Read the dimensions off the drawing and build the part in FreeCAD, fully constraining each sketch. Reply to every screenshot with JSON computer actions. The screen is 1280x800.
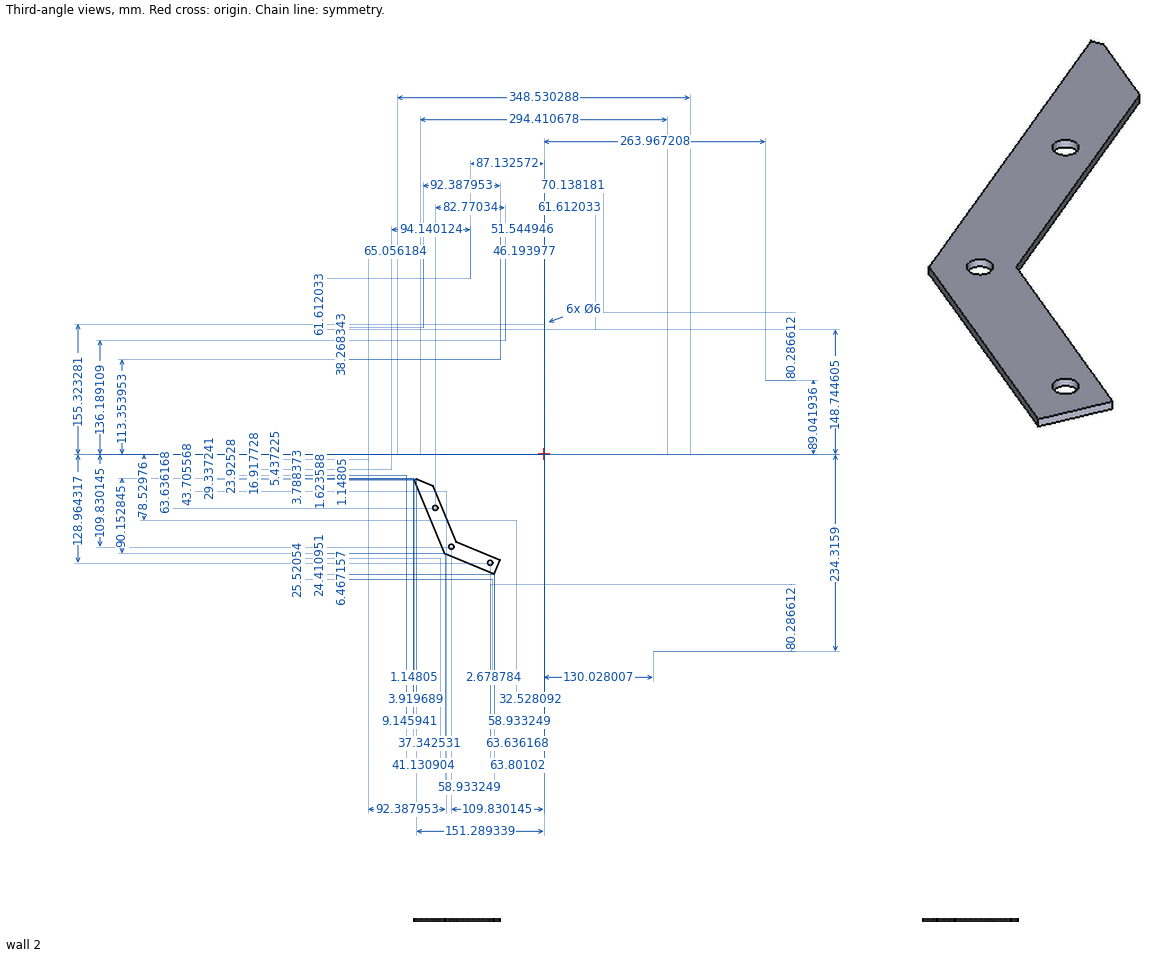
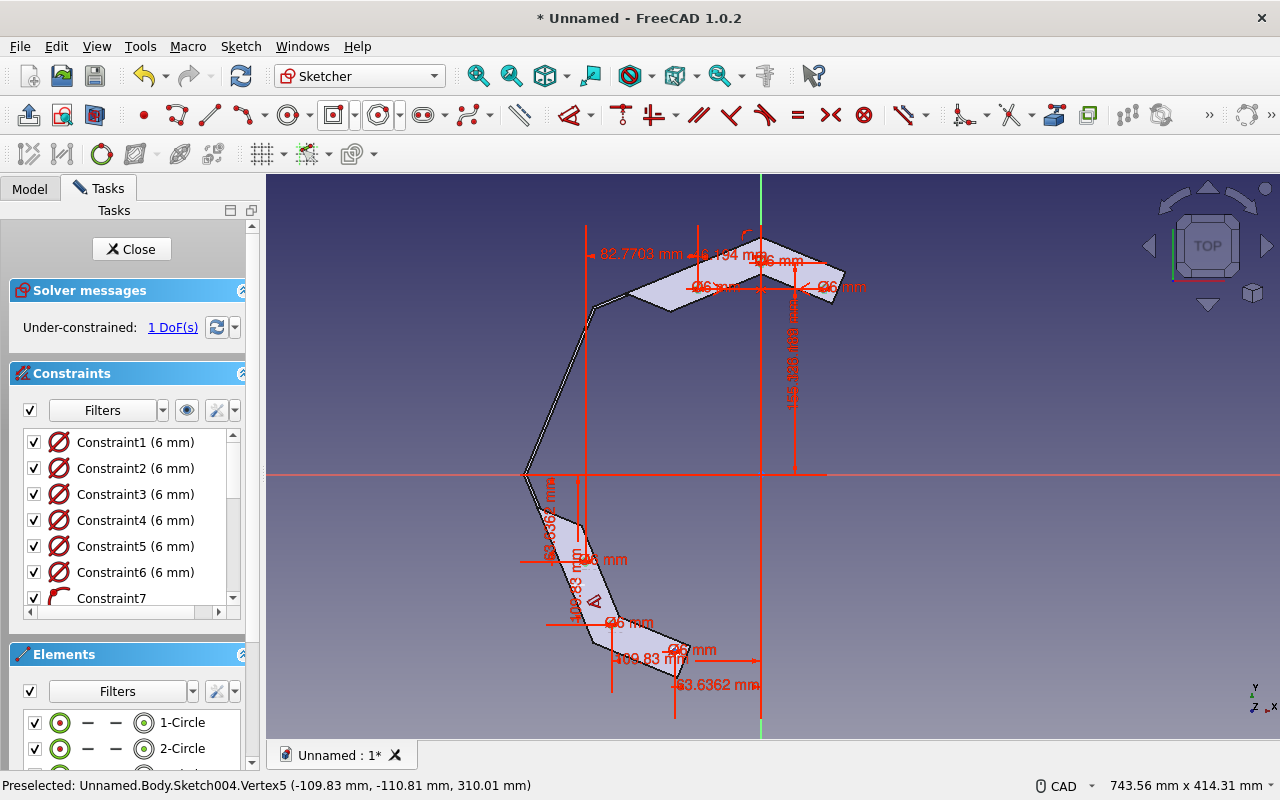
{"action": "left_click", "coordinate": [675, 652]}
{"action": "left_click", "coordinate": [795, 563]}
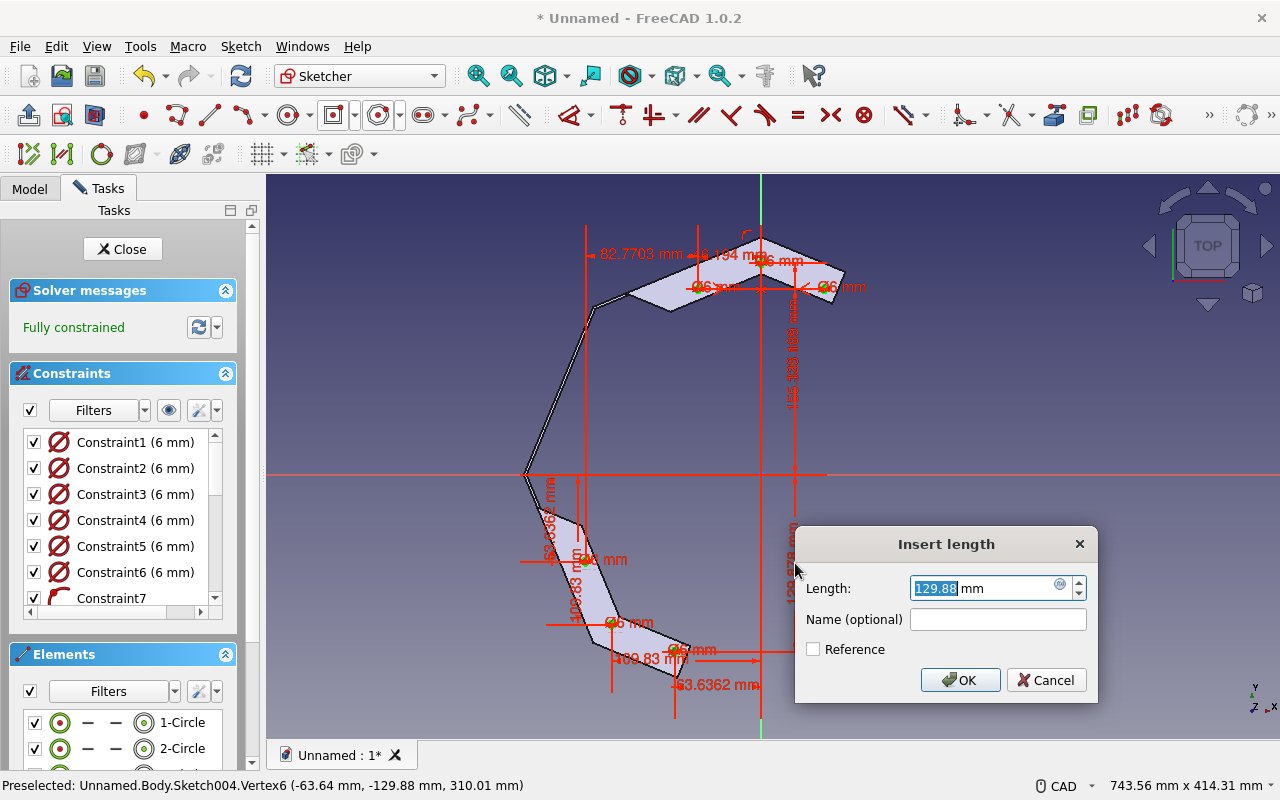
{"action": "type", "text": "128.964317"}
{"action": "key", "text": "Return"}
{"action": "key", "text": "Escape"}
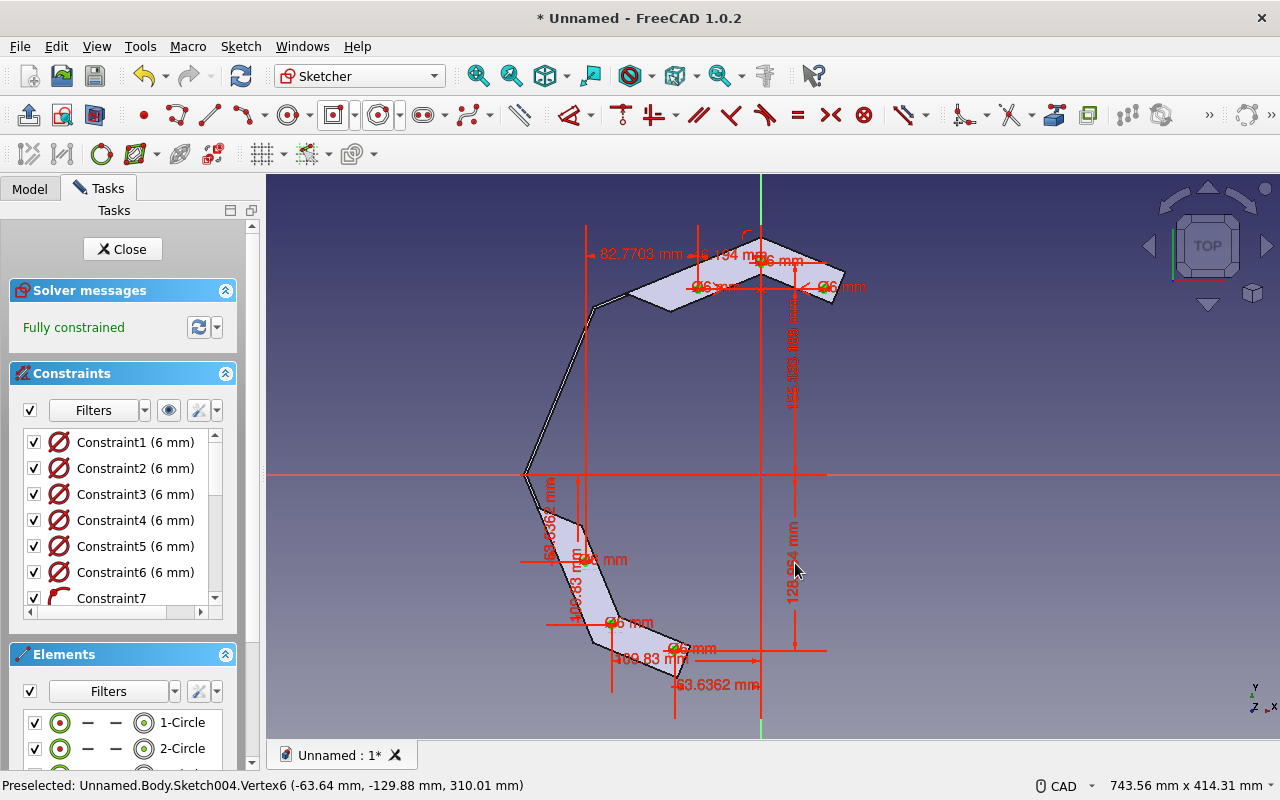
{"action": "left_click", "coordinate": [123, 249]}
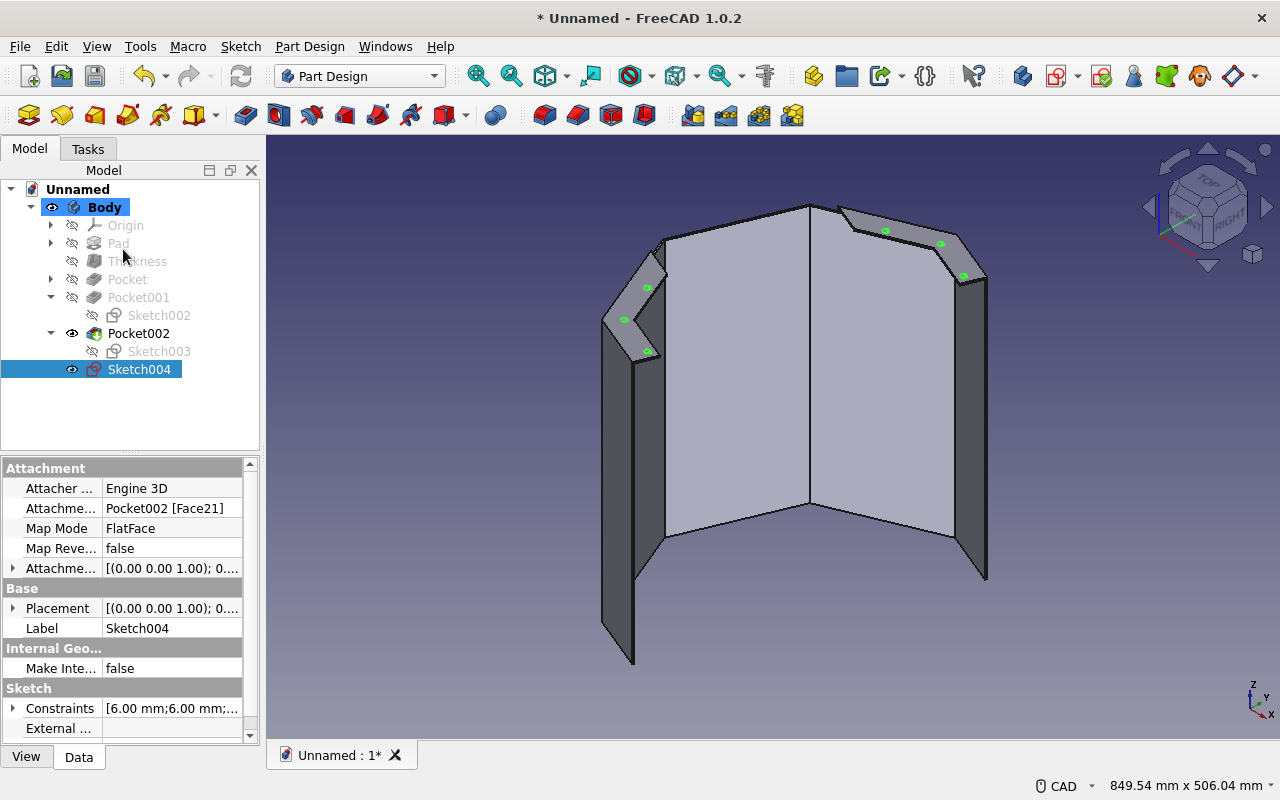
{"action": "left_click", "coordinate": [246, 116]}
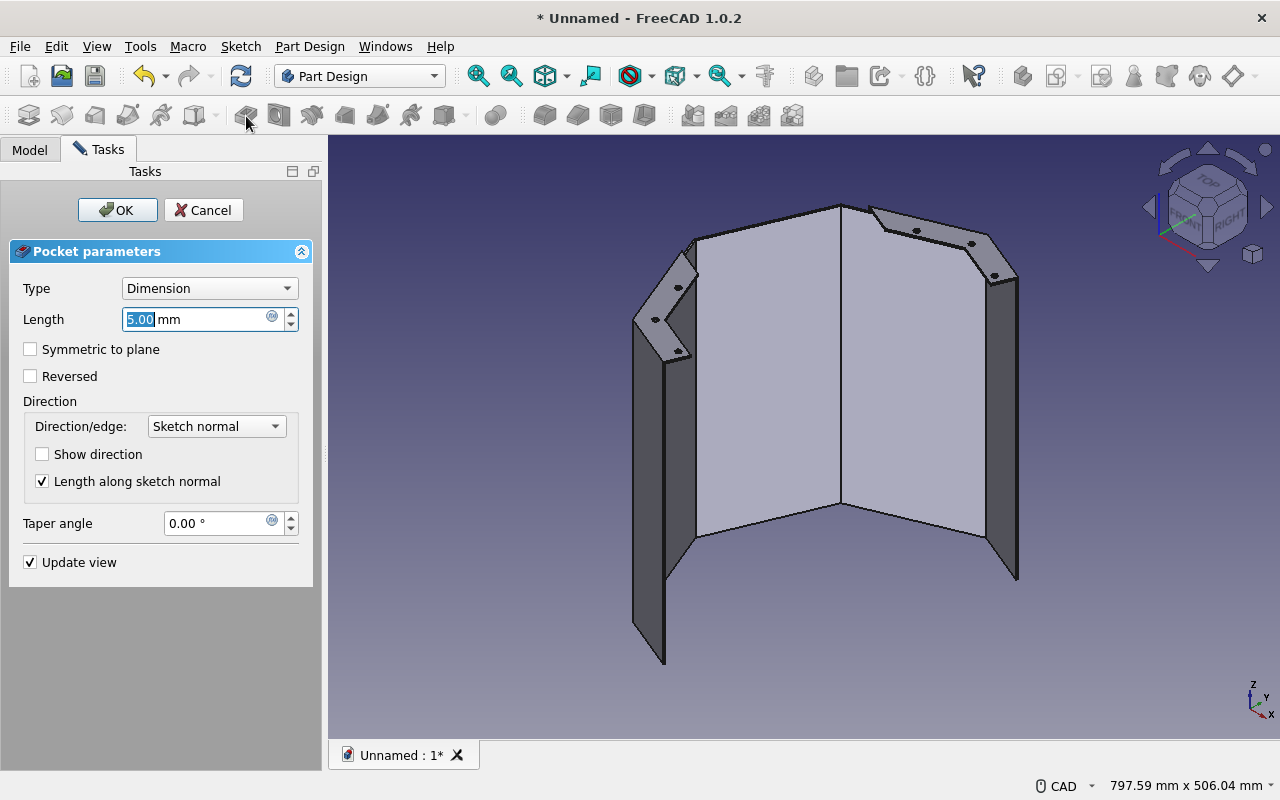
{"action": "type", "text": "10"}
{"action": "key", "text": "Tab"}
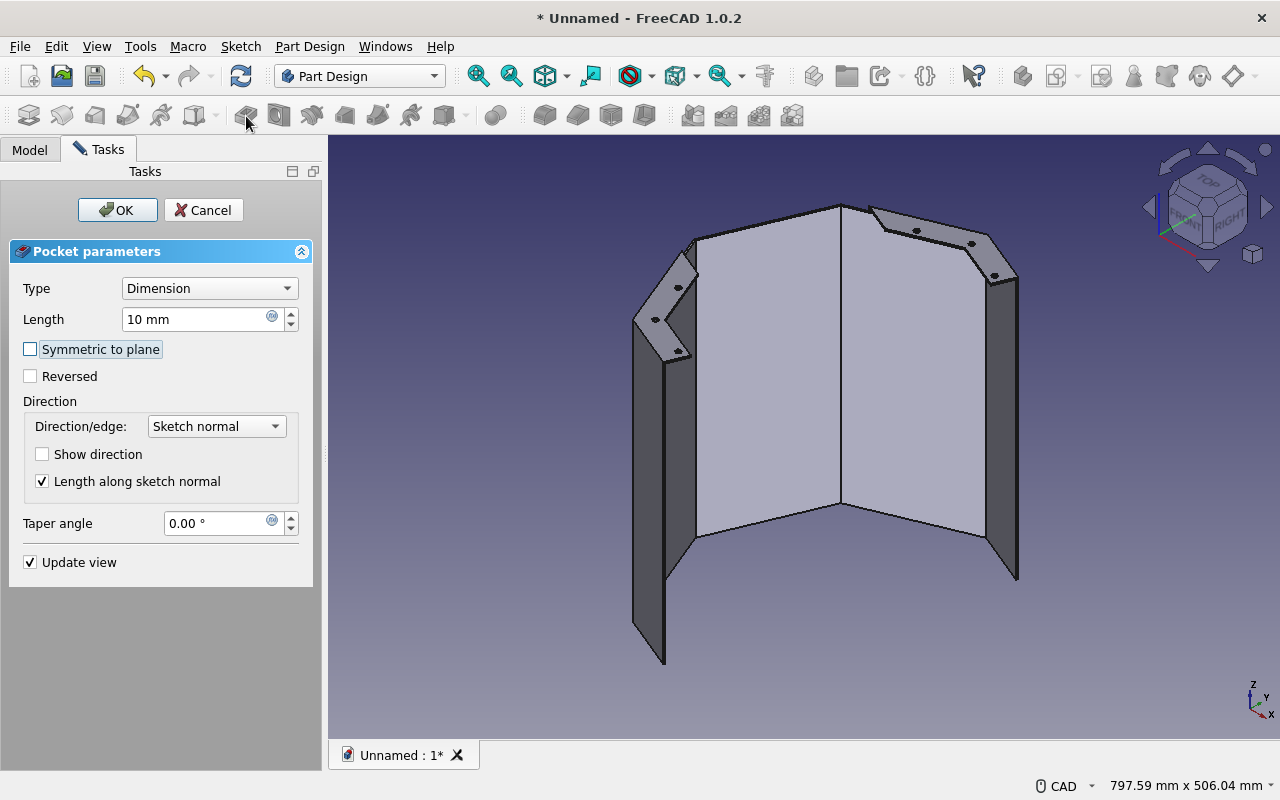
{"action": "left_click", "coordinate": [118, 210]}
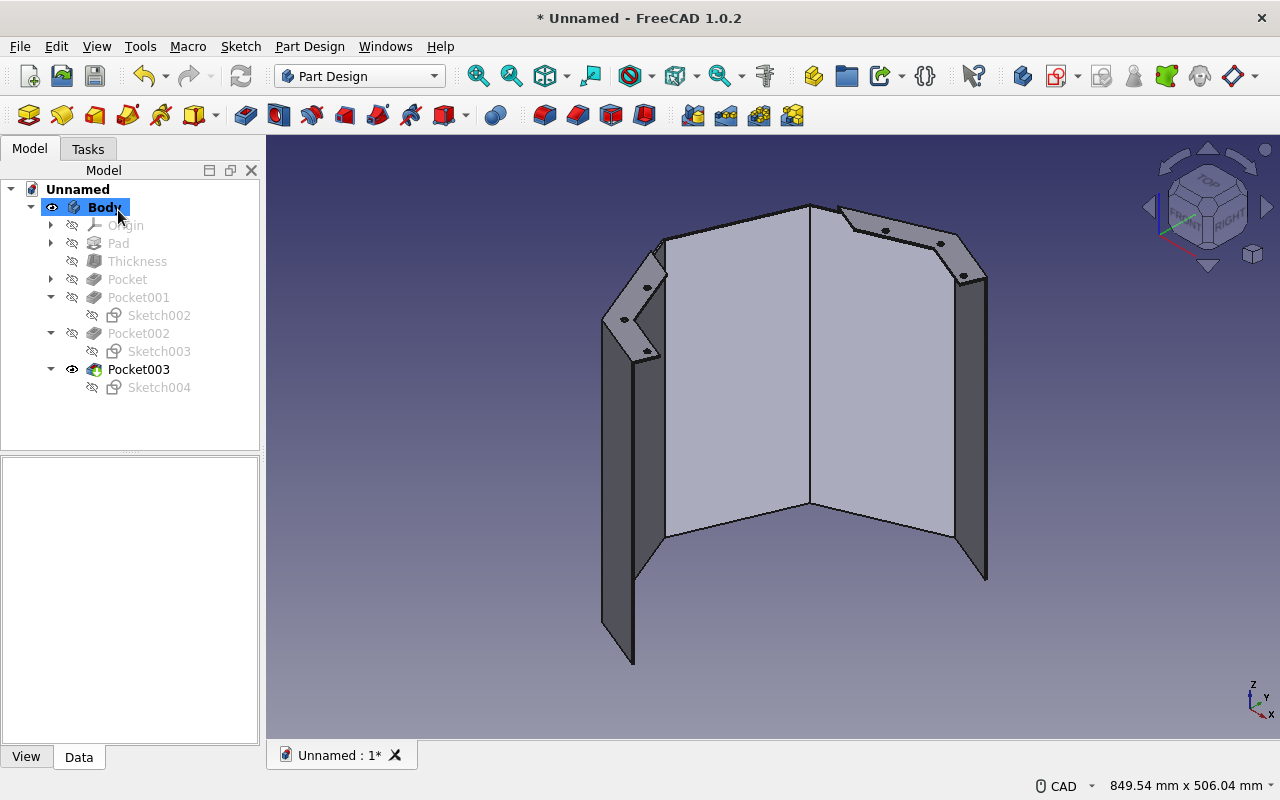
{"action": "left_click", "coordinate": [924, 234]}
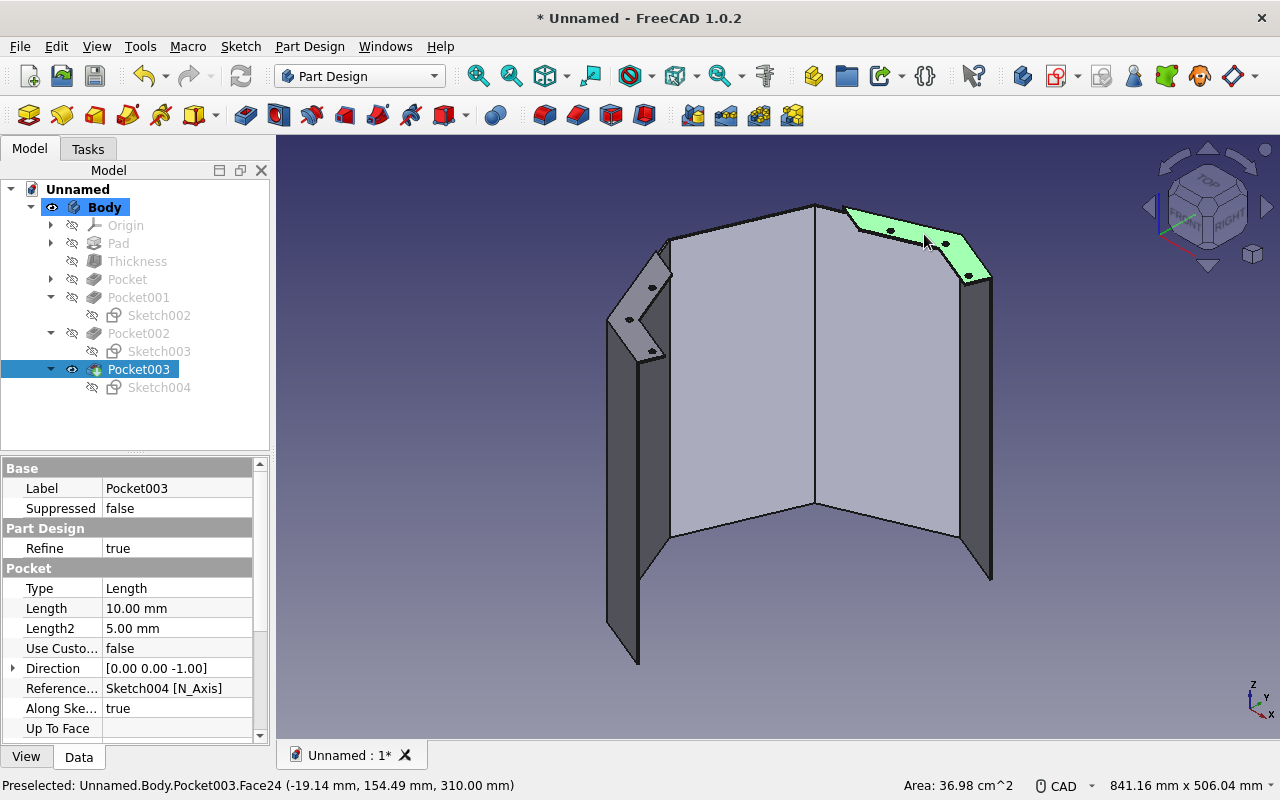
{"action": "left_click", "coordinate": [1056, 76]}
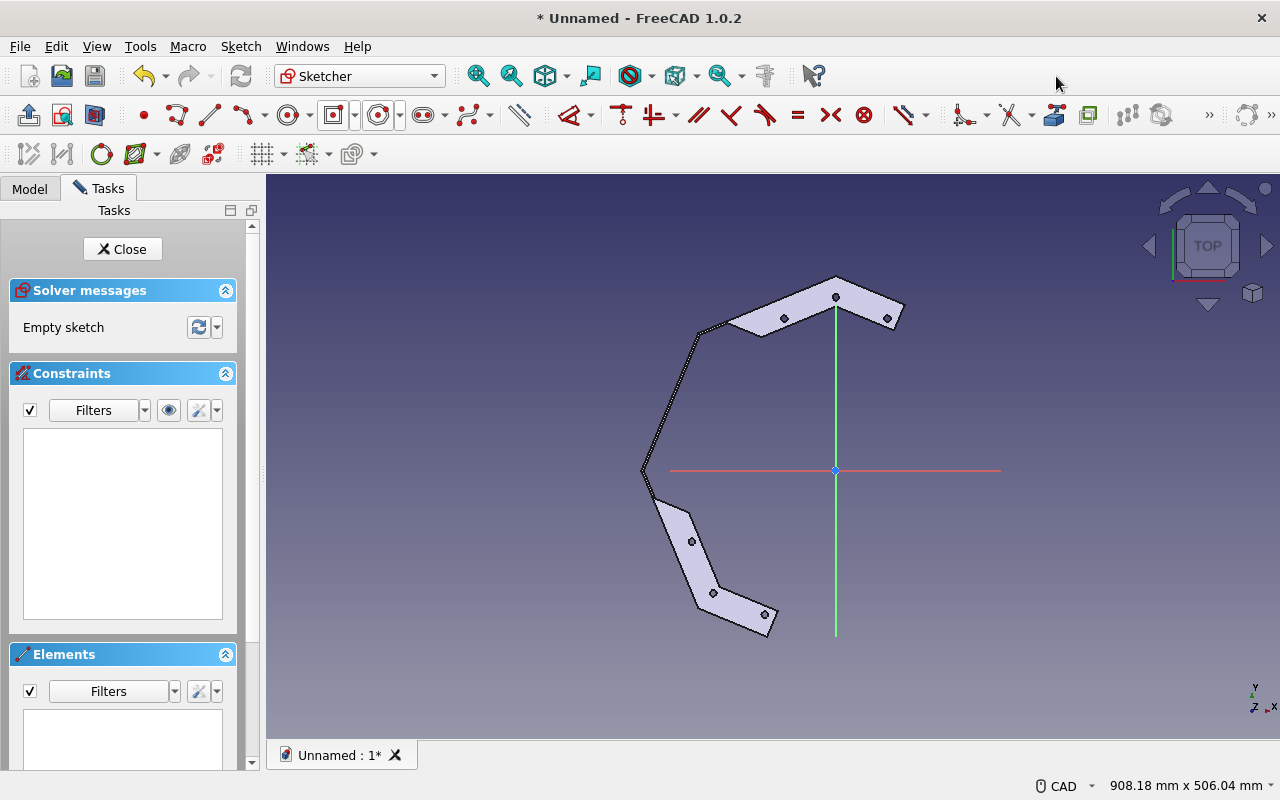
{"action": "left_click", "coordinate": [177, 116]}